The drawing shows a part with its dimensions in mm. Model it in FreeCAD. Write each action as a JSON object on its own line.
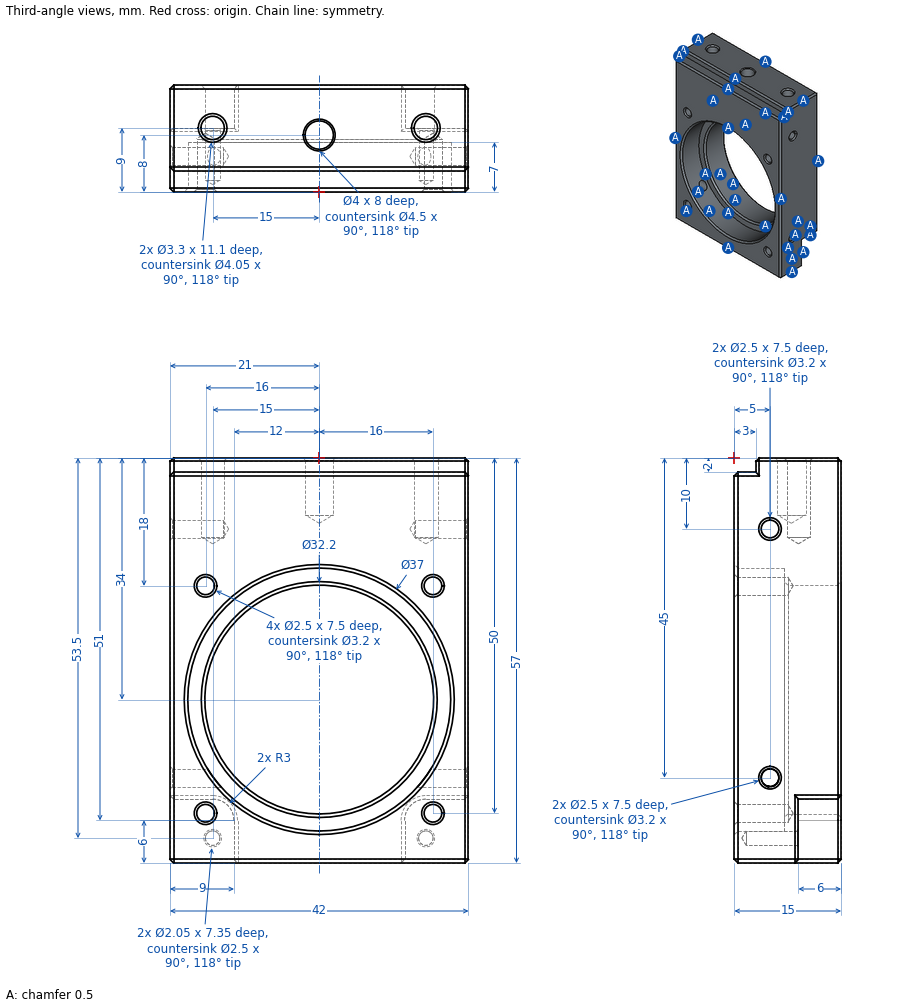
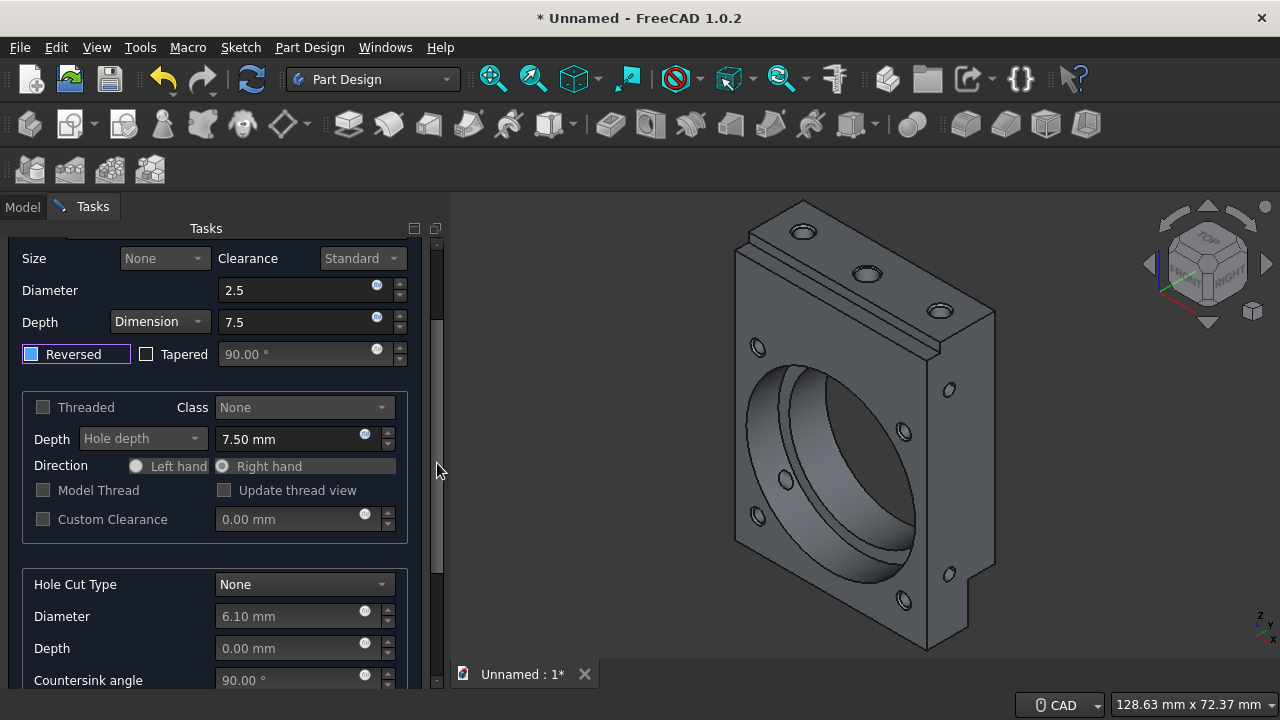
{"action": "left_click", "coordinate": [306, 584]}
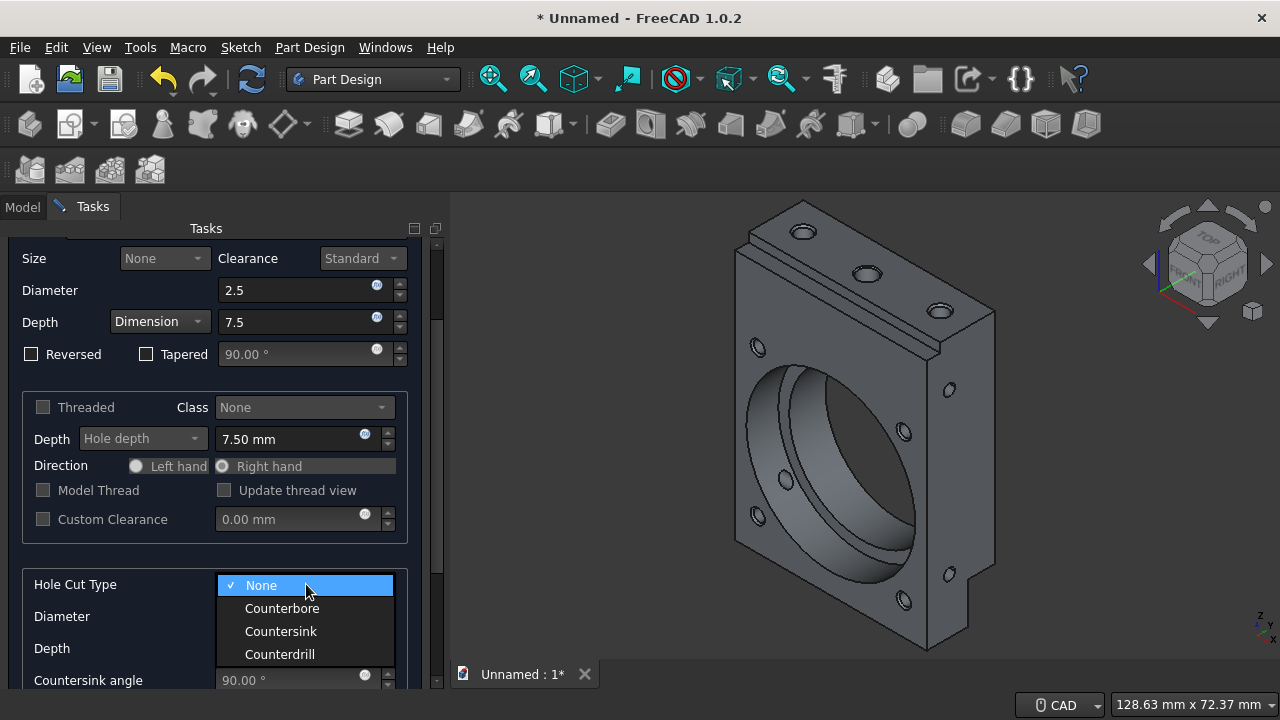
{"action": "left_click", "coordinate": [304, 632]}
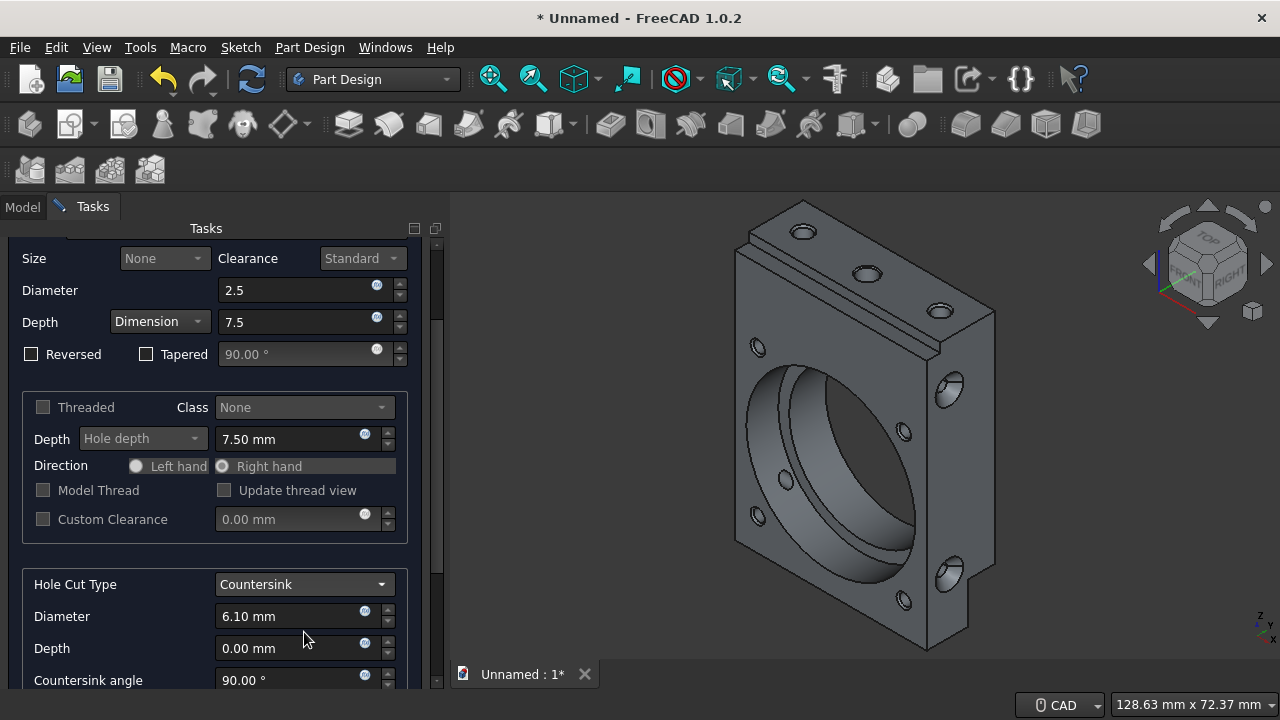
{"action": "triple_click", "coordinate": [298, 616]}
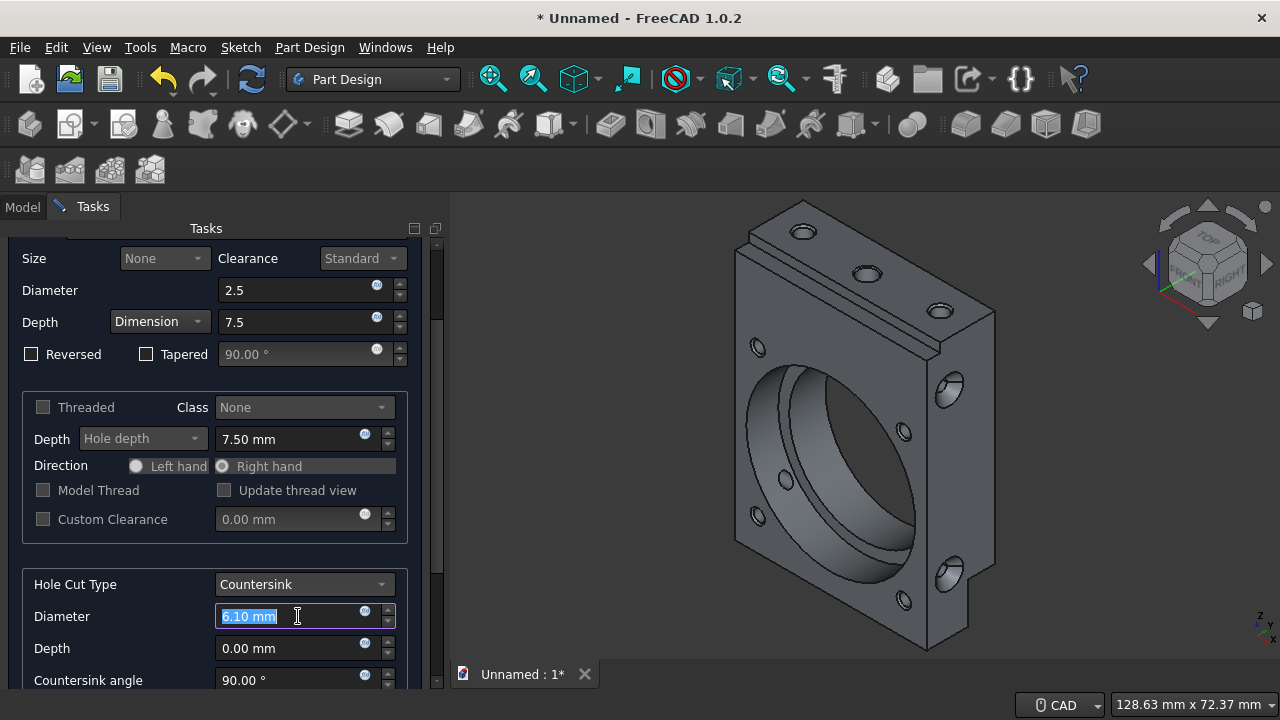
{"action": "type", "text": "3.2"}
{"action": "key", "text": "Tab"}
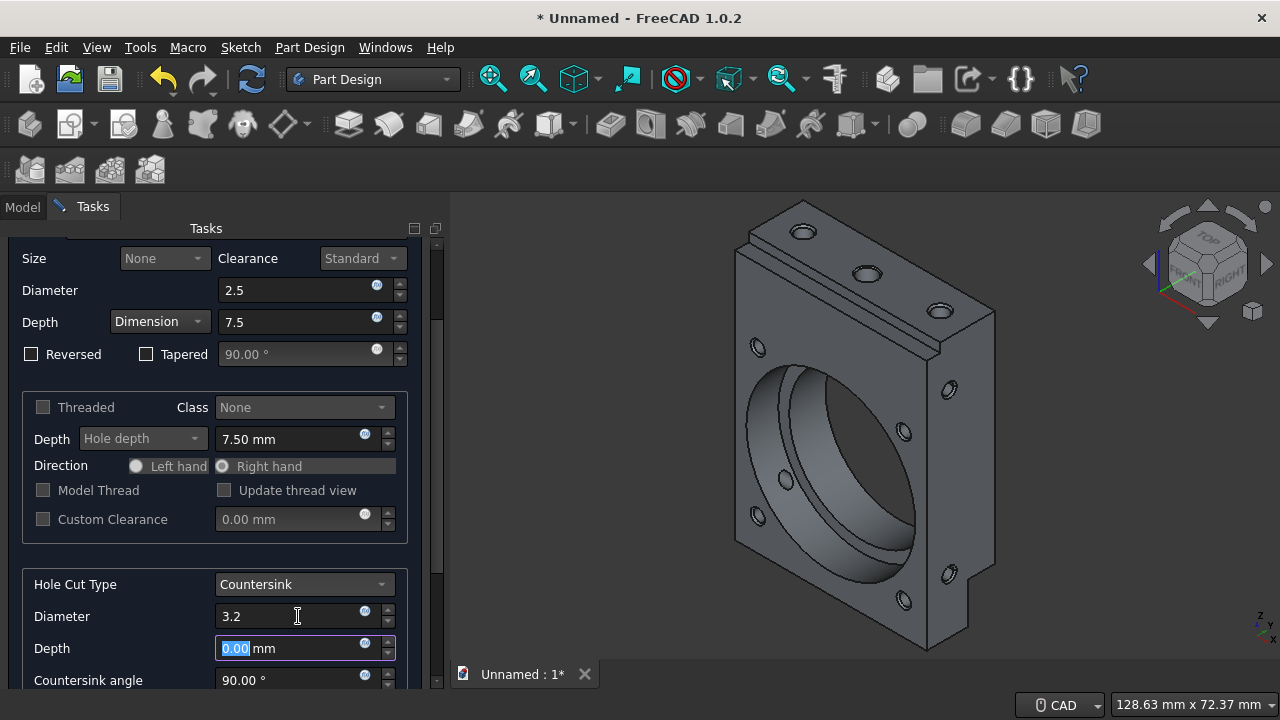
{"action": "scroll", "coordinate": [437, 463], "scroll_direction": "up", "scroll_amount": 3}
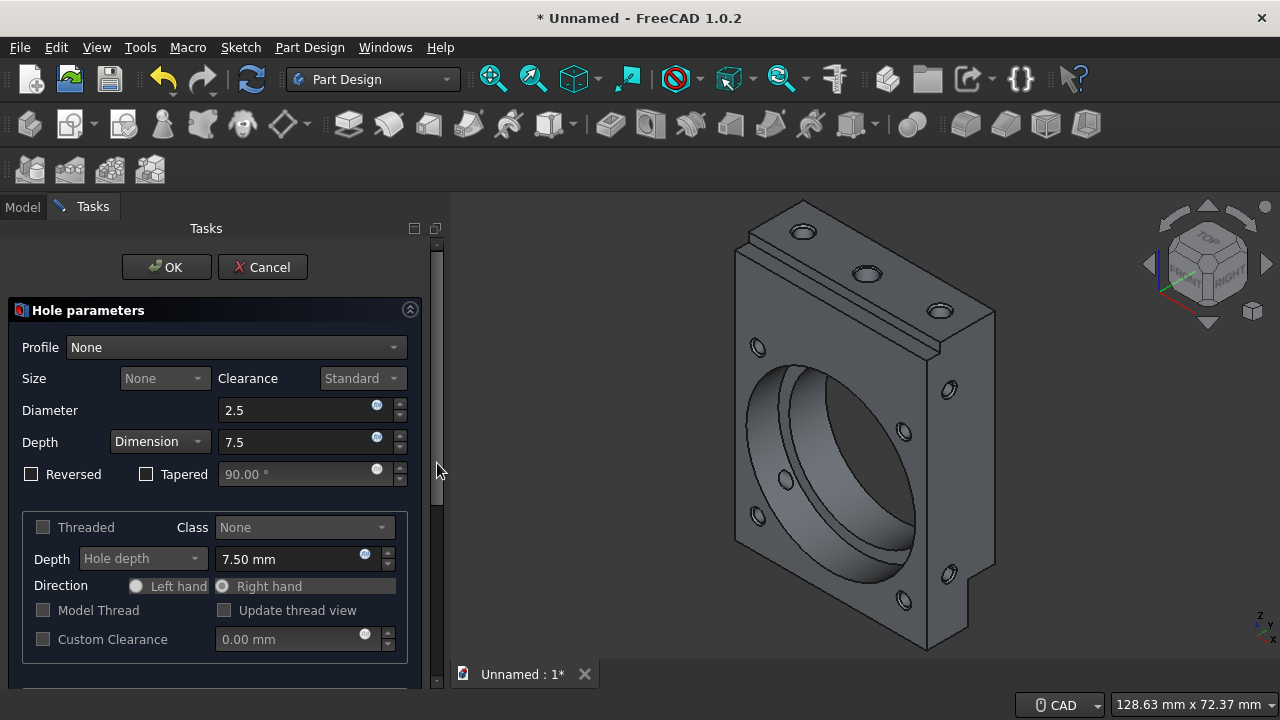
{"action": "left_click", "coordinate": [167, 267]}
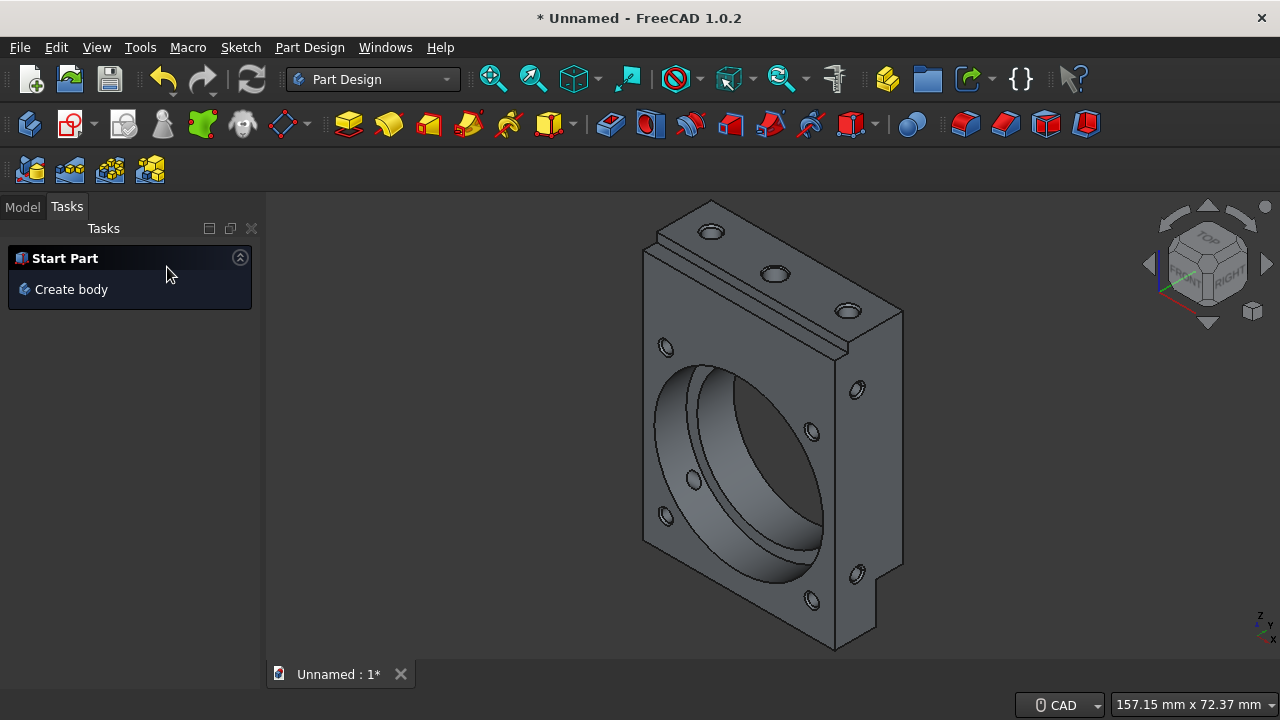
{"action": "left_click", "coordinate": [654, 425]}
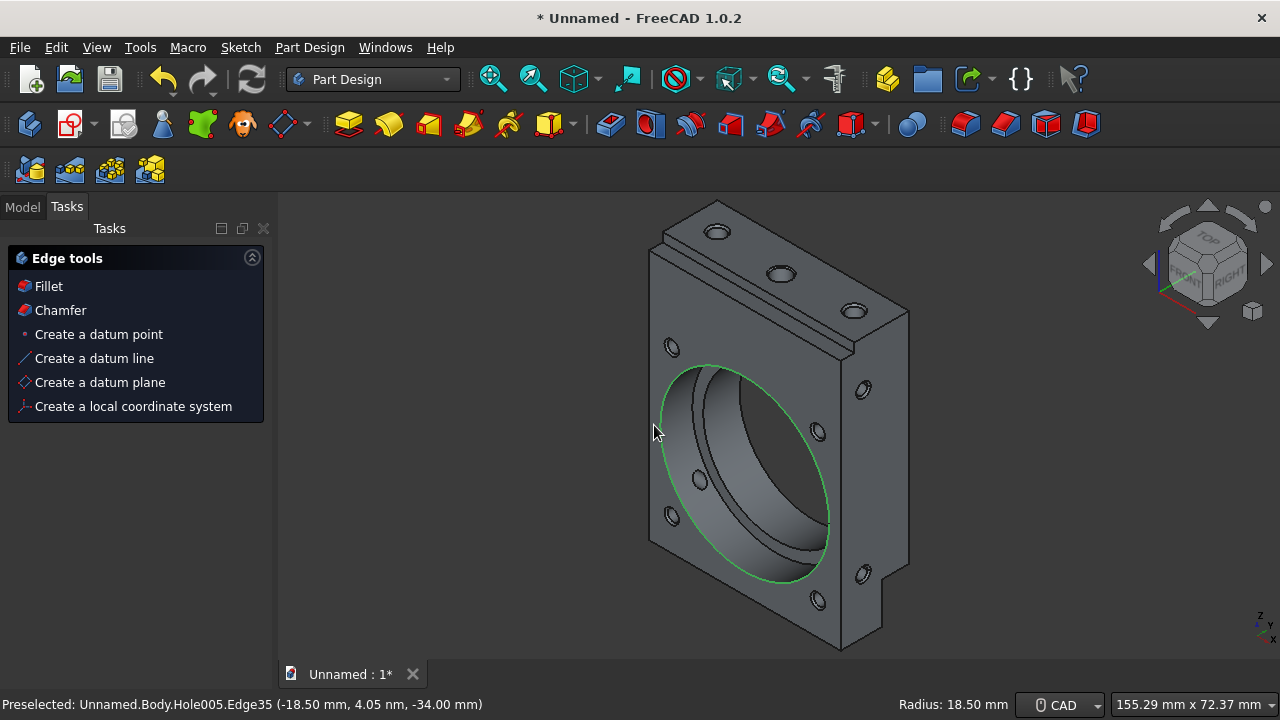
{"action": "left_click", "coordinate": [703, 412], "text": "ctrl"}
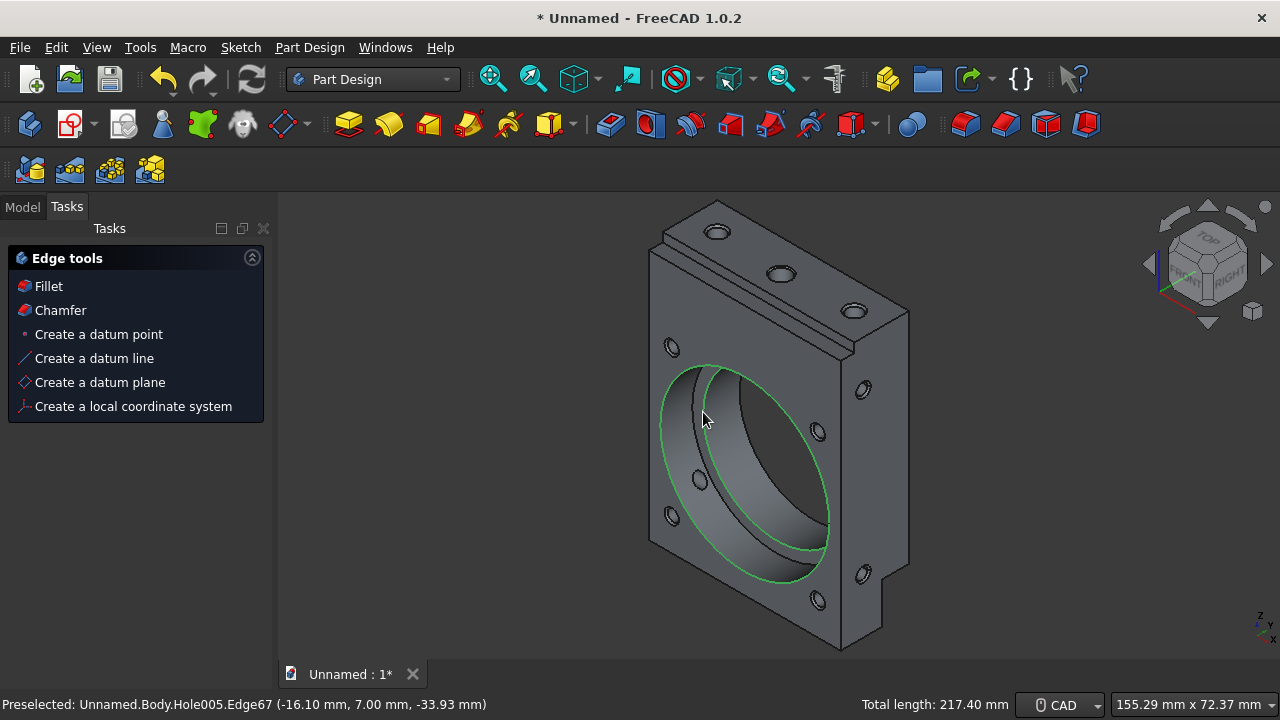
{"action": "left_click", "coordinate": [841, 505], "text": "ctrl"}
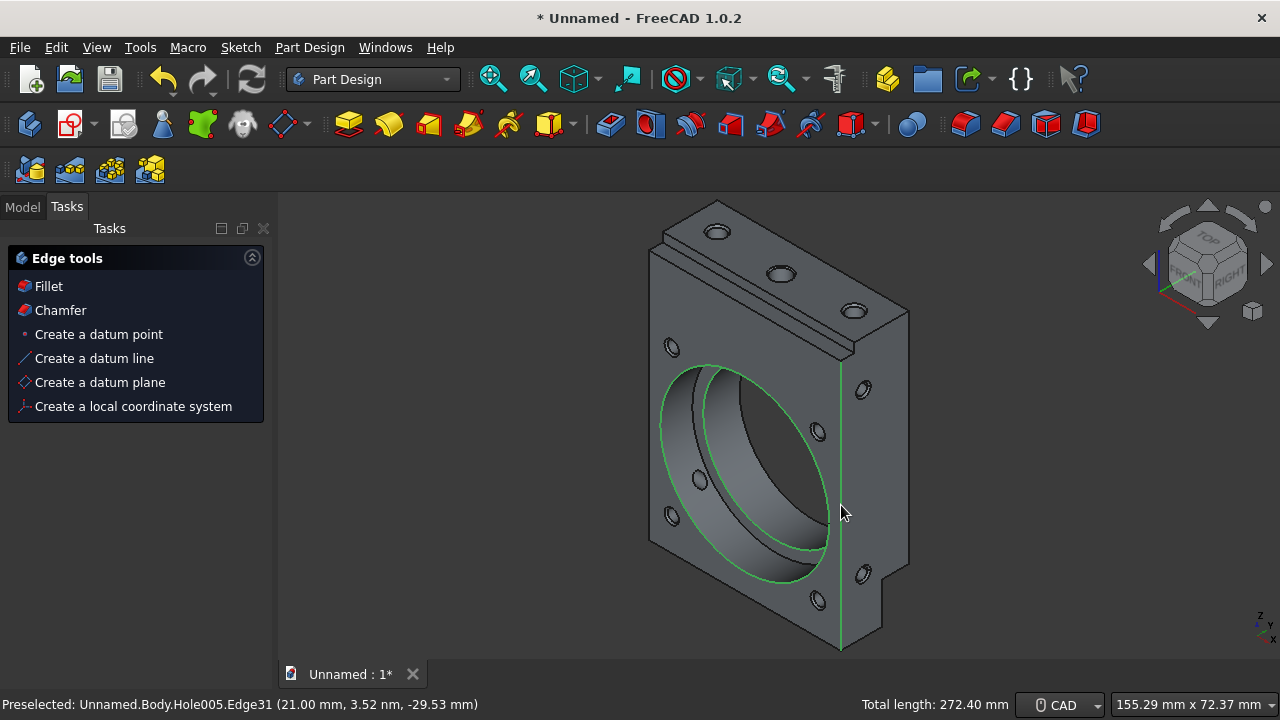
{"action": "left_click", "coordinate": [758, 286], "text": "ctrl"}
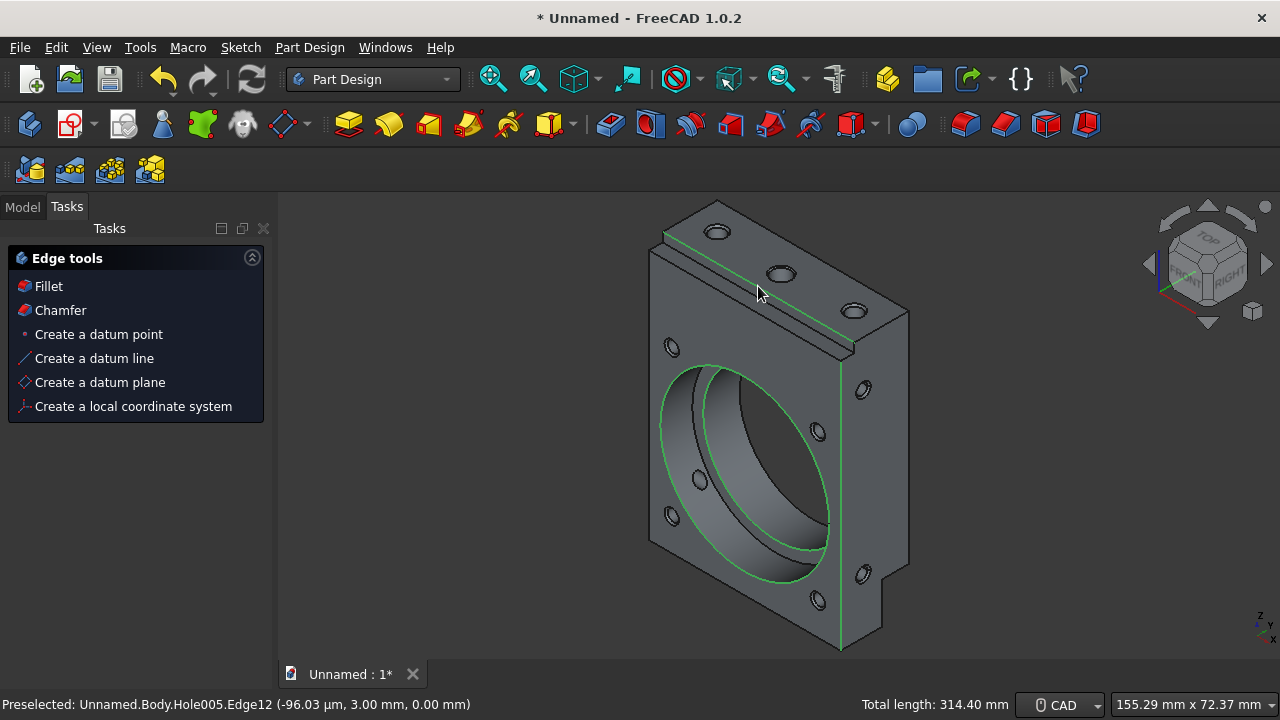
{"action": "left_click", "coordinate": [745, 305], "text": "ctrl"}